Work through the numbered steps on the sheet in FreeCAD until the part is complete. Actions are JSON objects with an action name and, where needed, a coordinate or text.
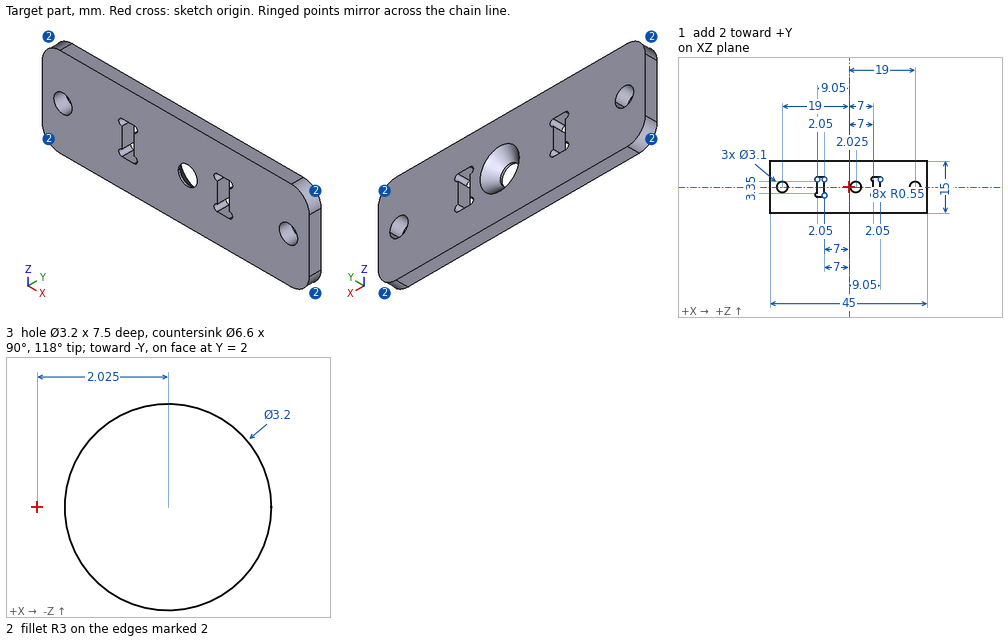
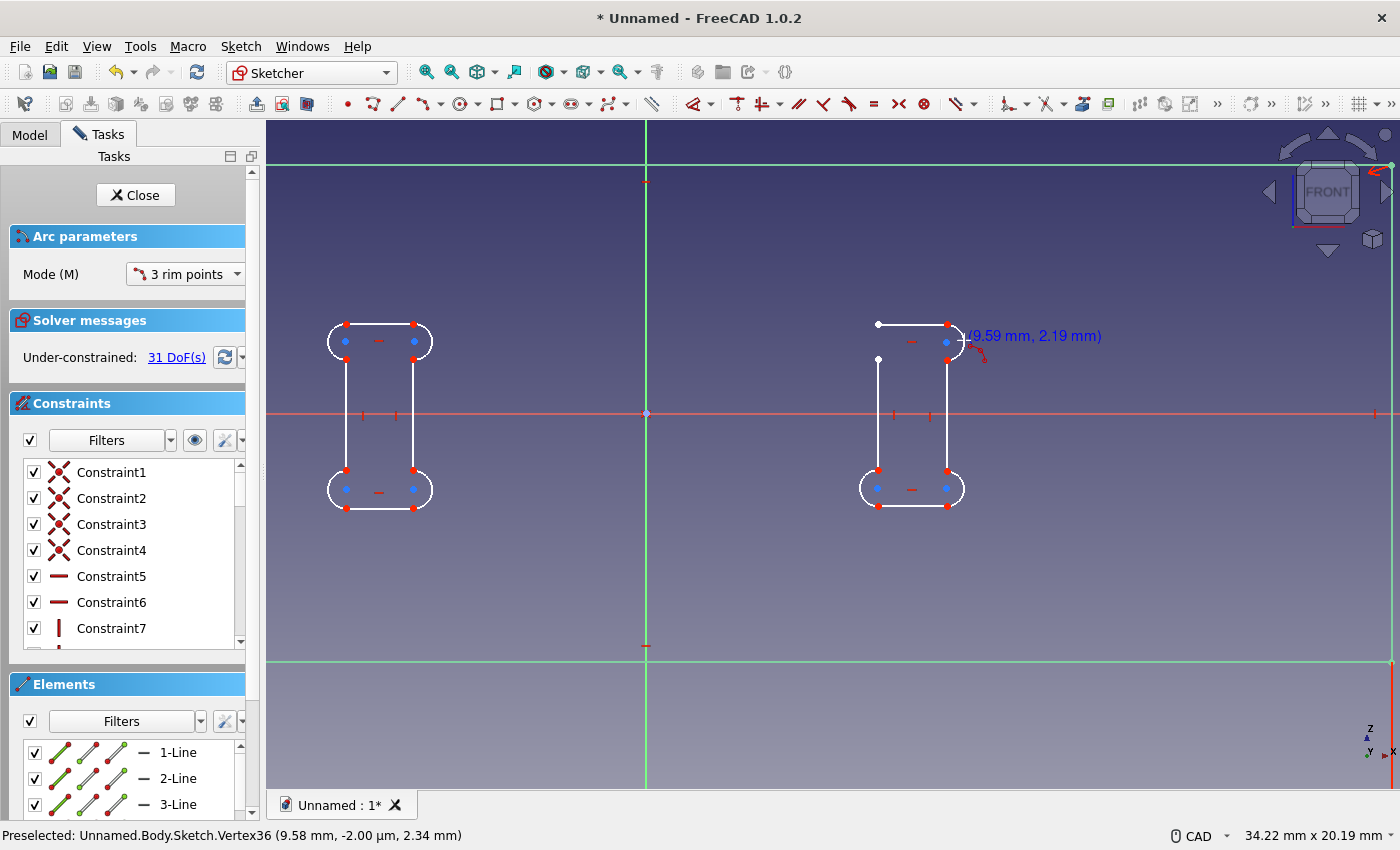
{"action": "left_click", "coordinate": [878, 325]}
{"action": "left_click", "coordinate": [878, 359]}
{"action": "left_click", "coordinate": [860, 340]}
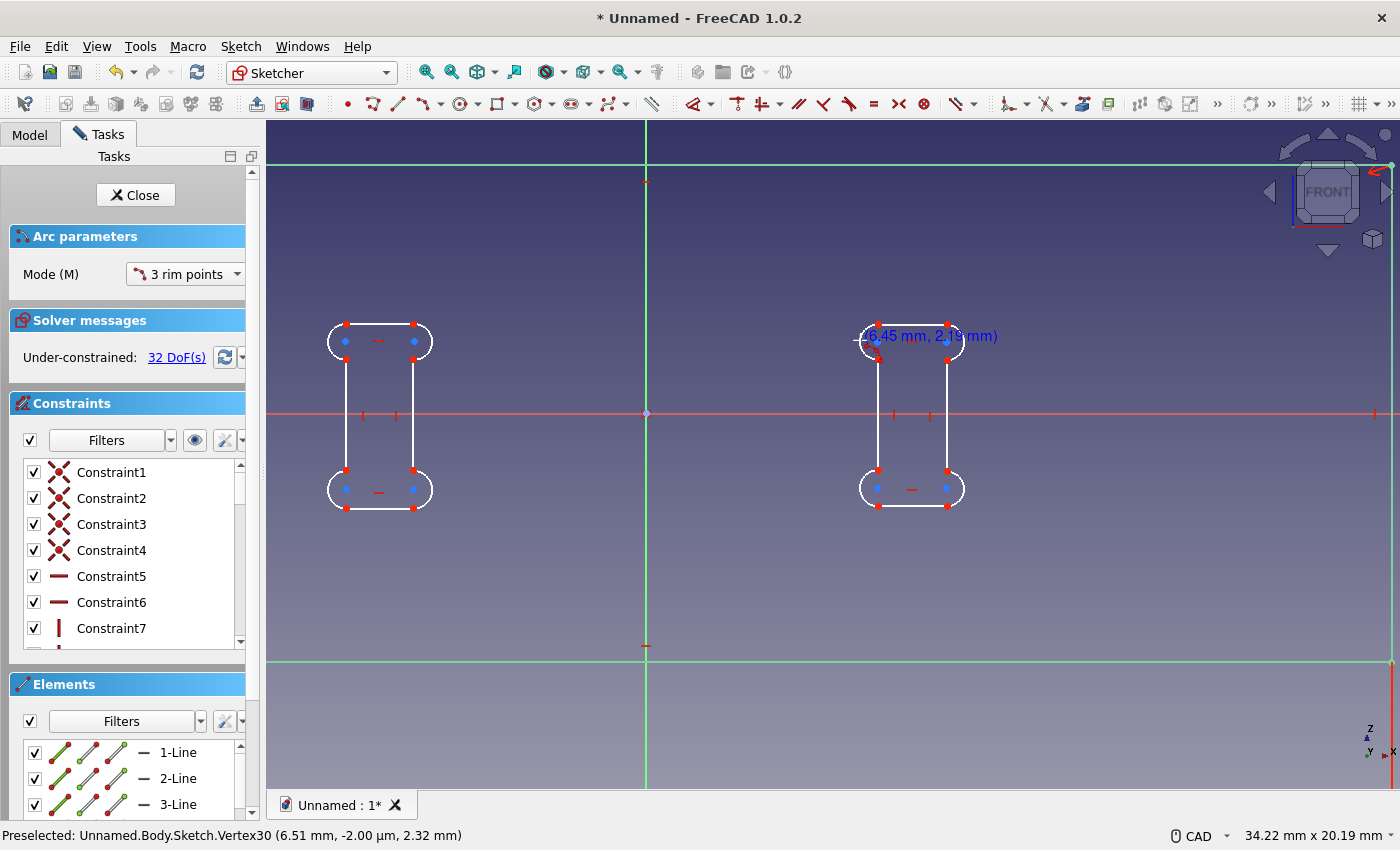
{"action": "left_click", "coordinate": [460, 104]}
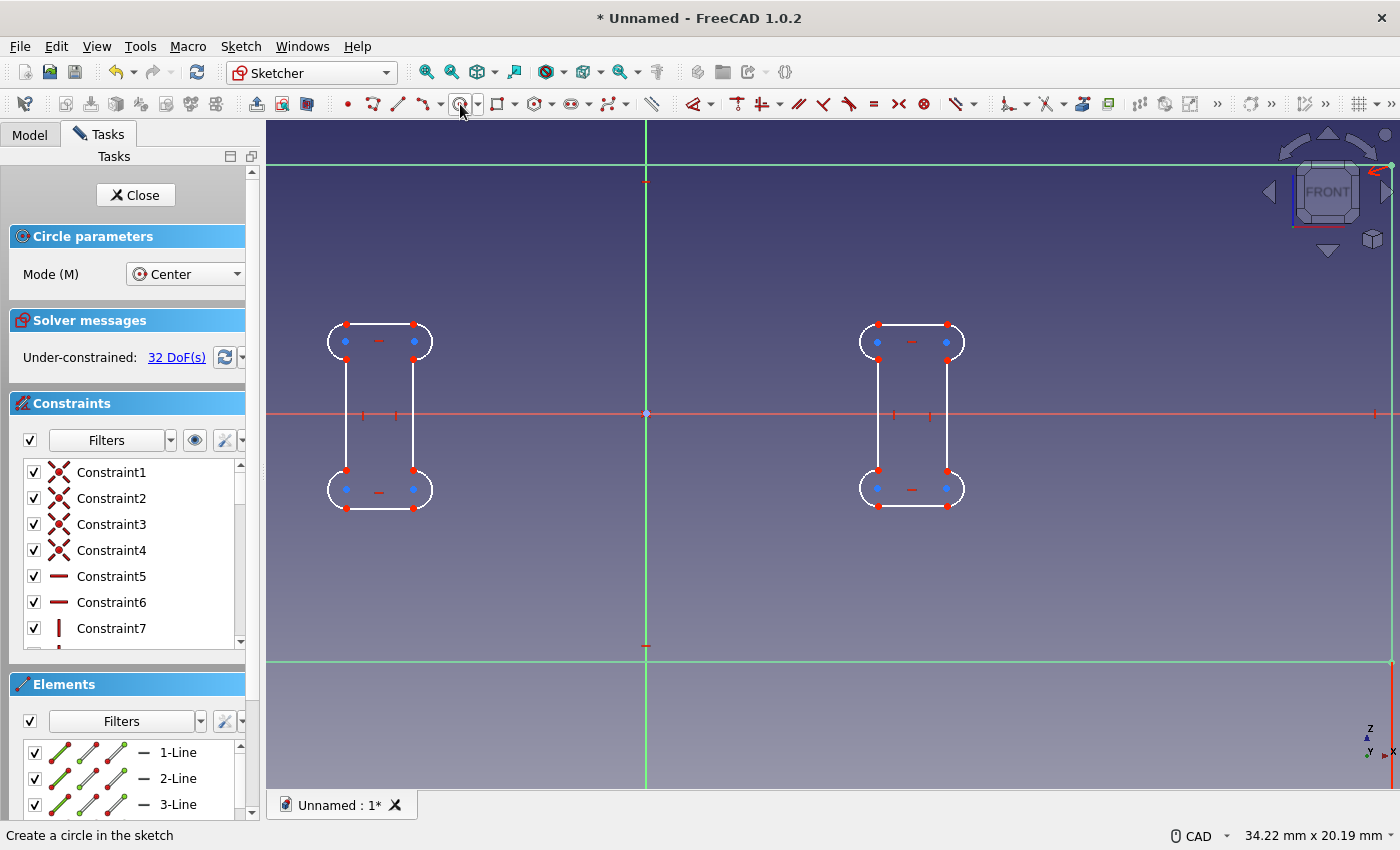
{"action": "scroll", "coordinate": [861, 488], "scroll_direction": "down", "scroll_amount": 4}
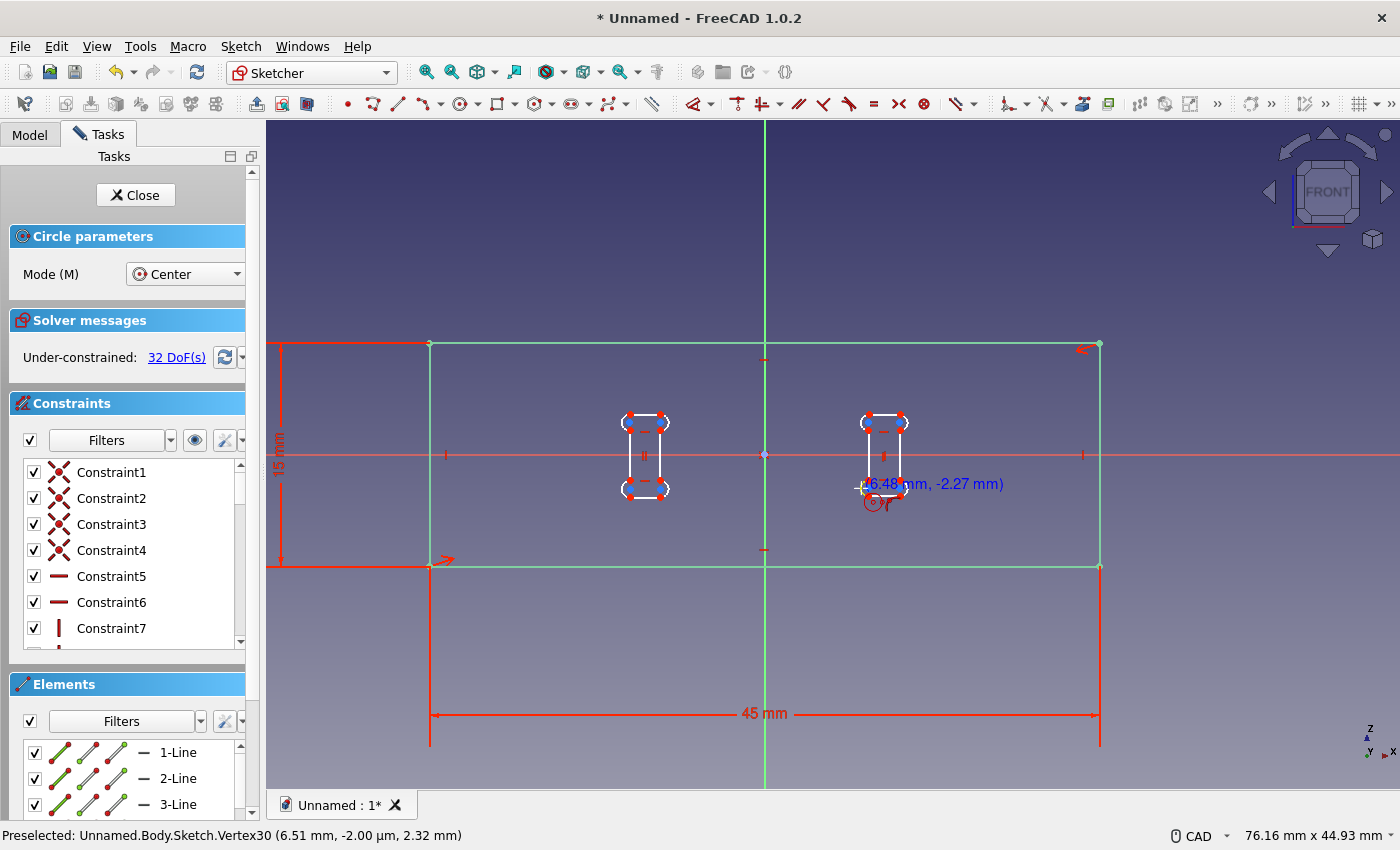
{"action": "left_click", "coordinate": [482, 455]}
{"action": "mouse_move", "coordinate": [498, 439]}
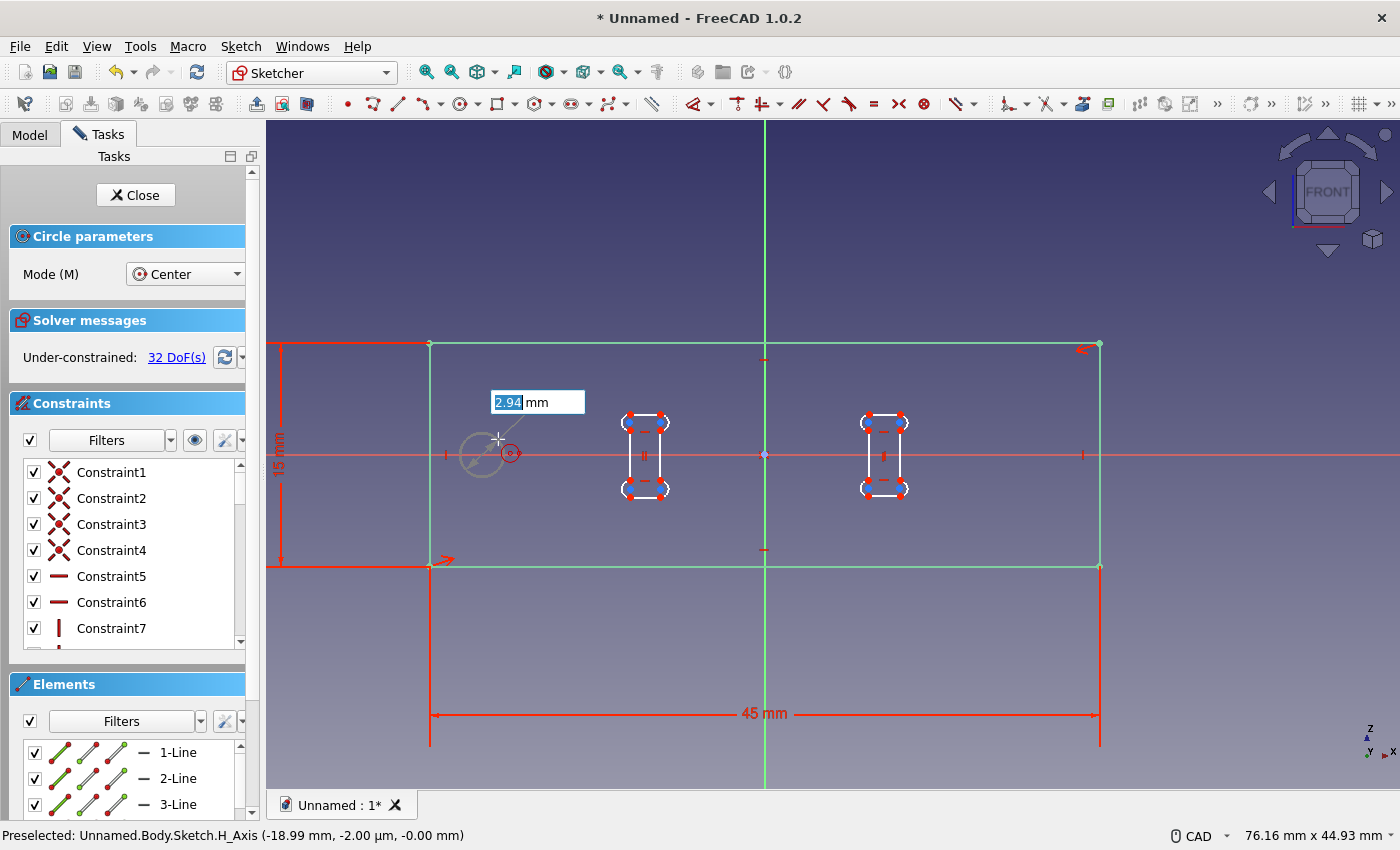
{"action": "type", "text": "3.1"}
{"action": "key", "text": "Return"}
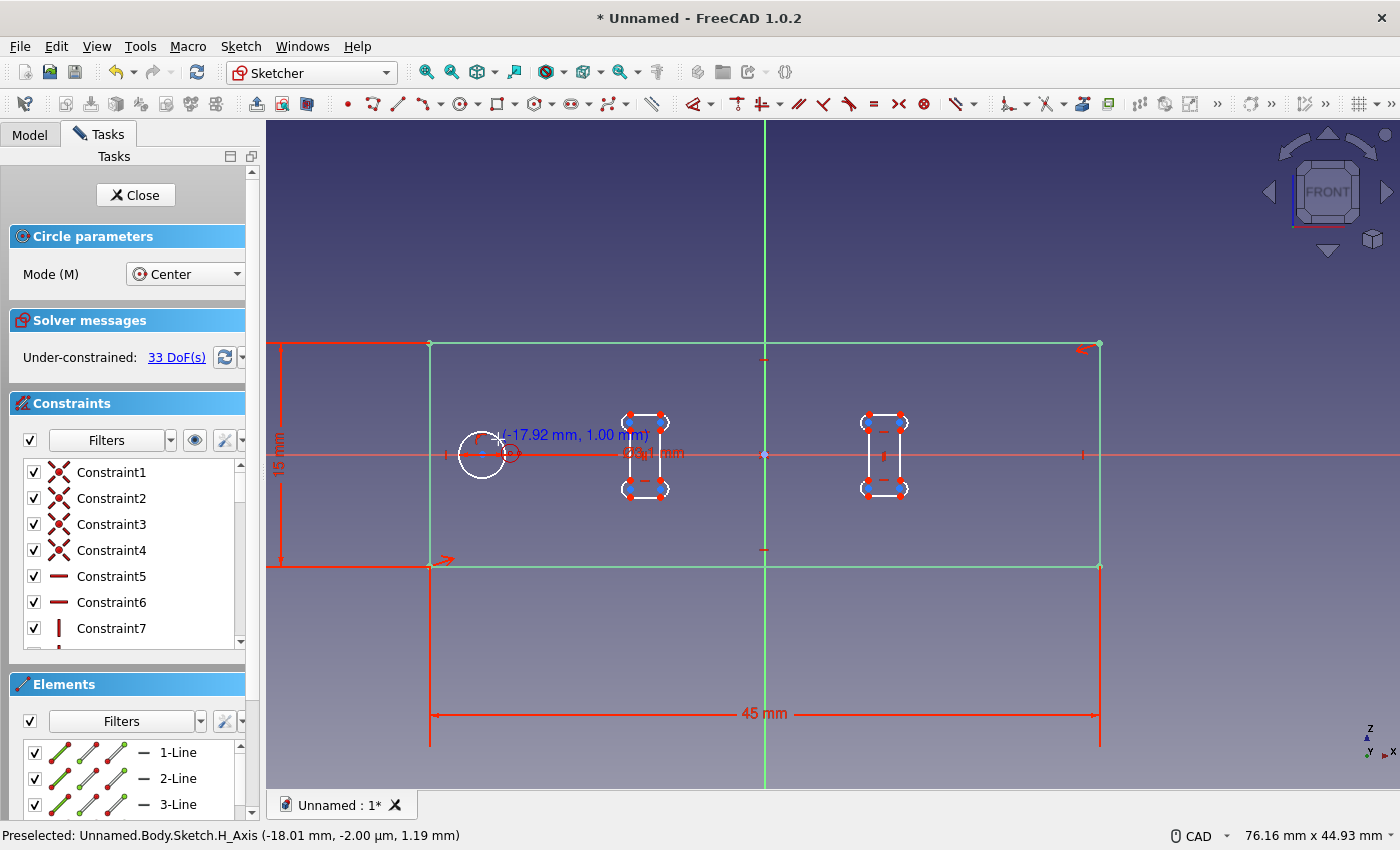
{"action": "left_click", "coordinate": [795, 455]}
{"action": "mouse_move", "coordinate": [811, 439]}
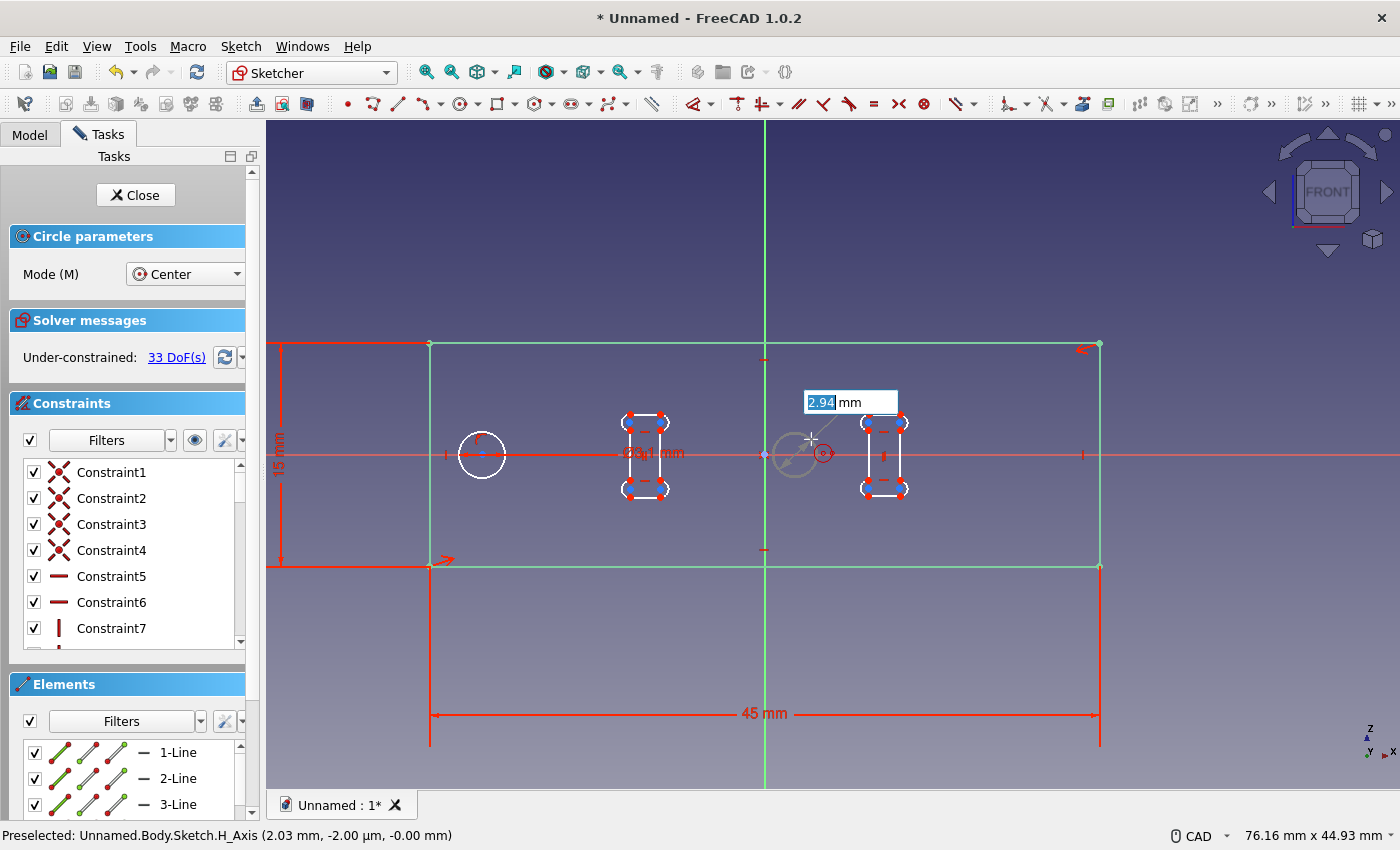
{"action": "type", "text": "3.1"}
{"action": "key", "text": "Return"}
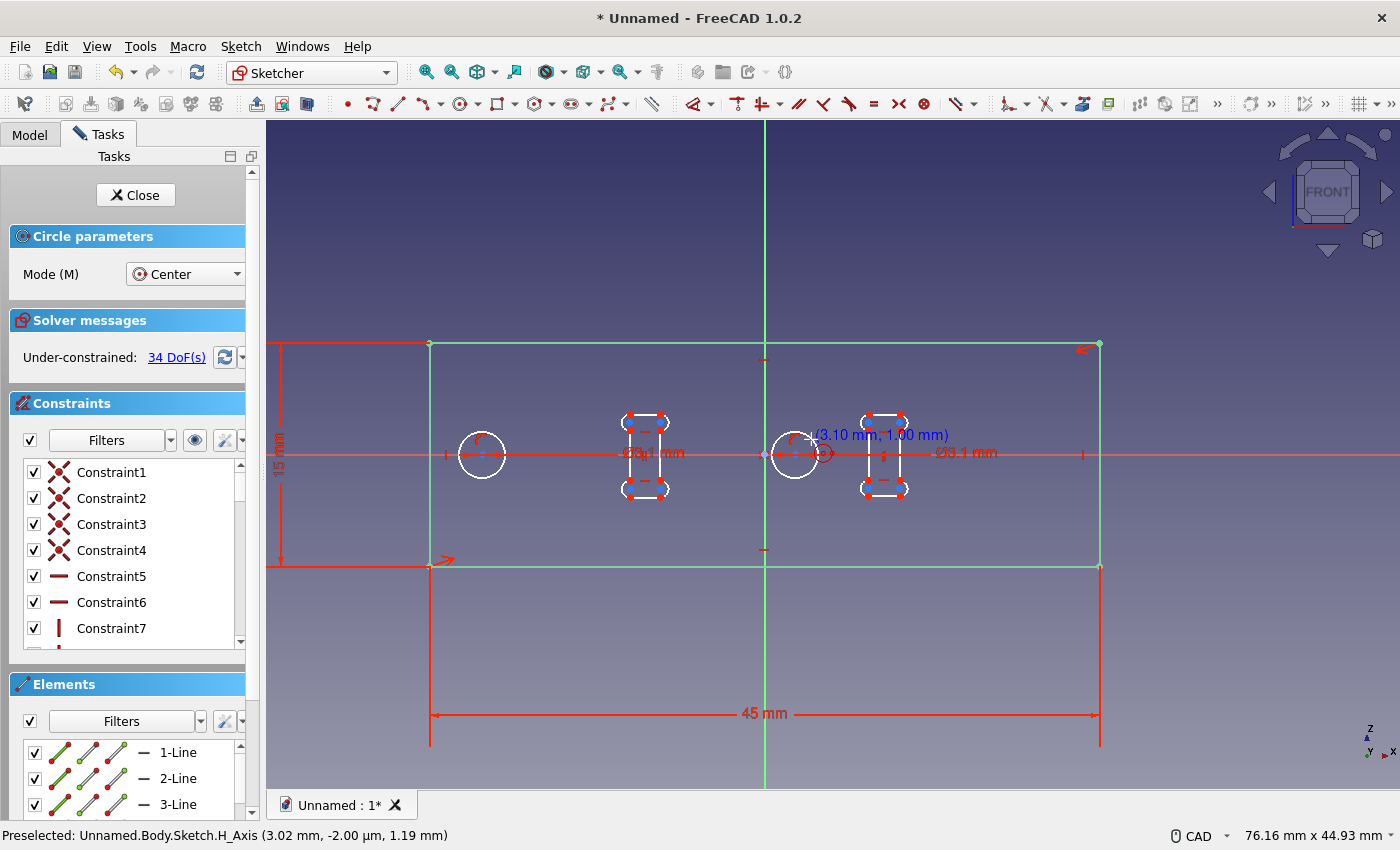
{"action": "left_click", "coordinate": [1048, 455]}
{"action": "mouse_move", "coordinate": [1064, 439]}